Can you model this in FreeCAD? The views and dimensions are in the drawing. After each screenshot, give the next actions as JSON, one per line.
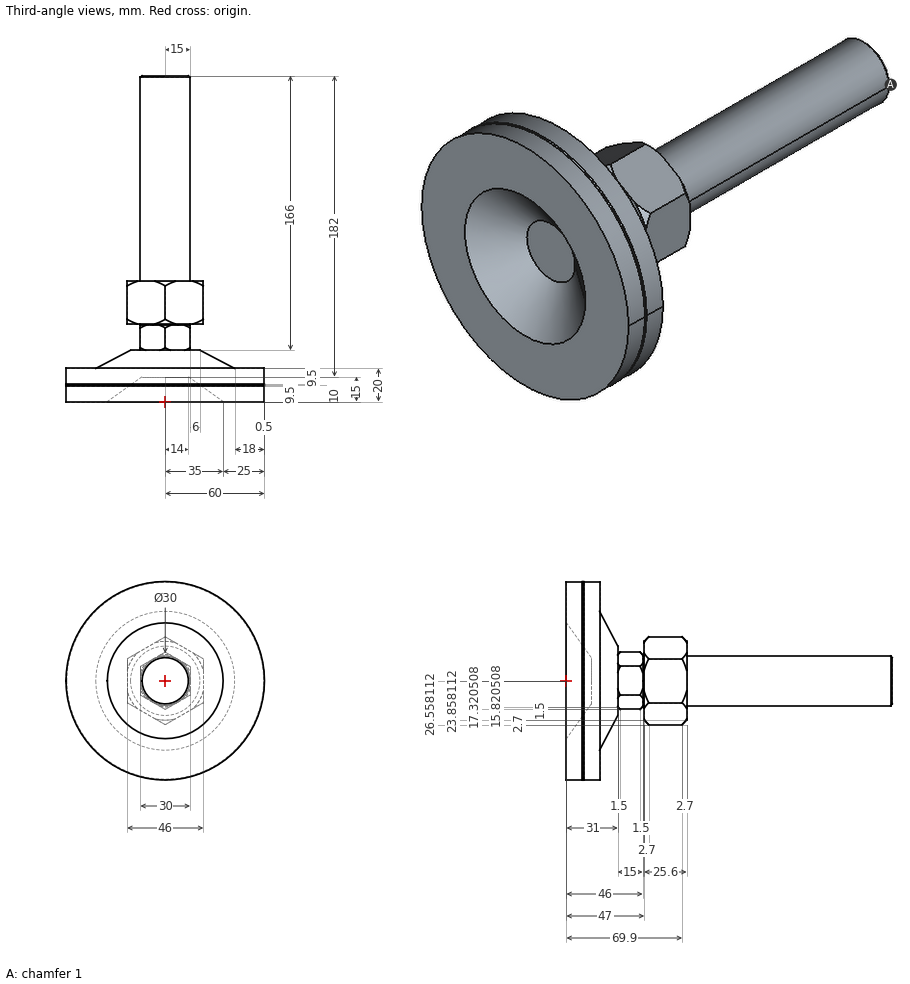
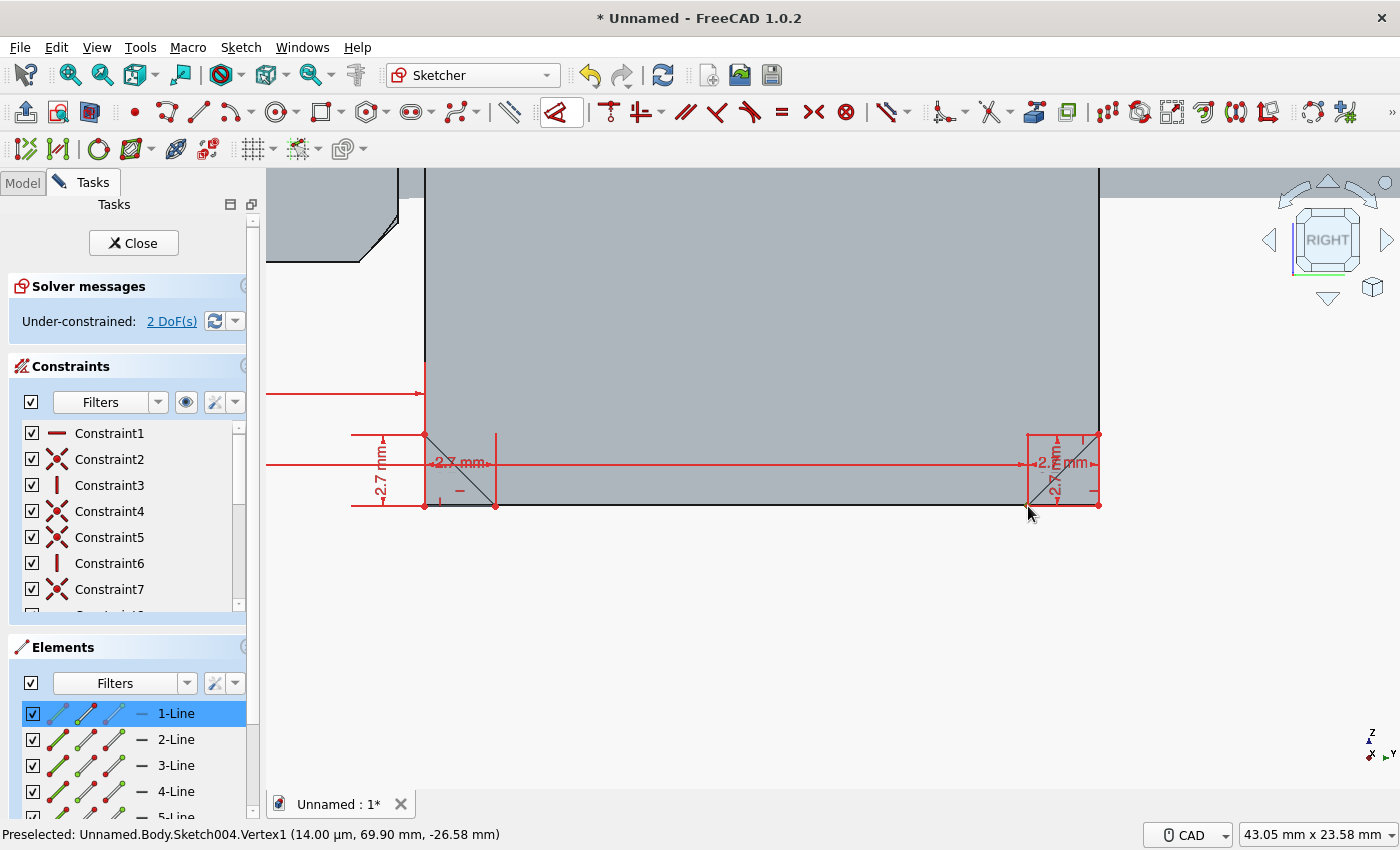
{"action": "key", "text": "i"}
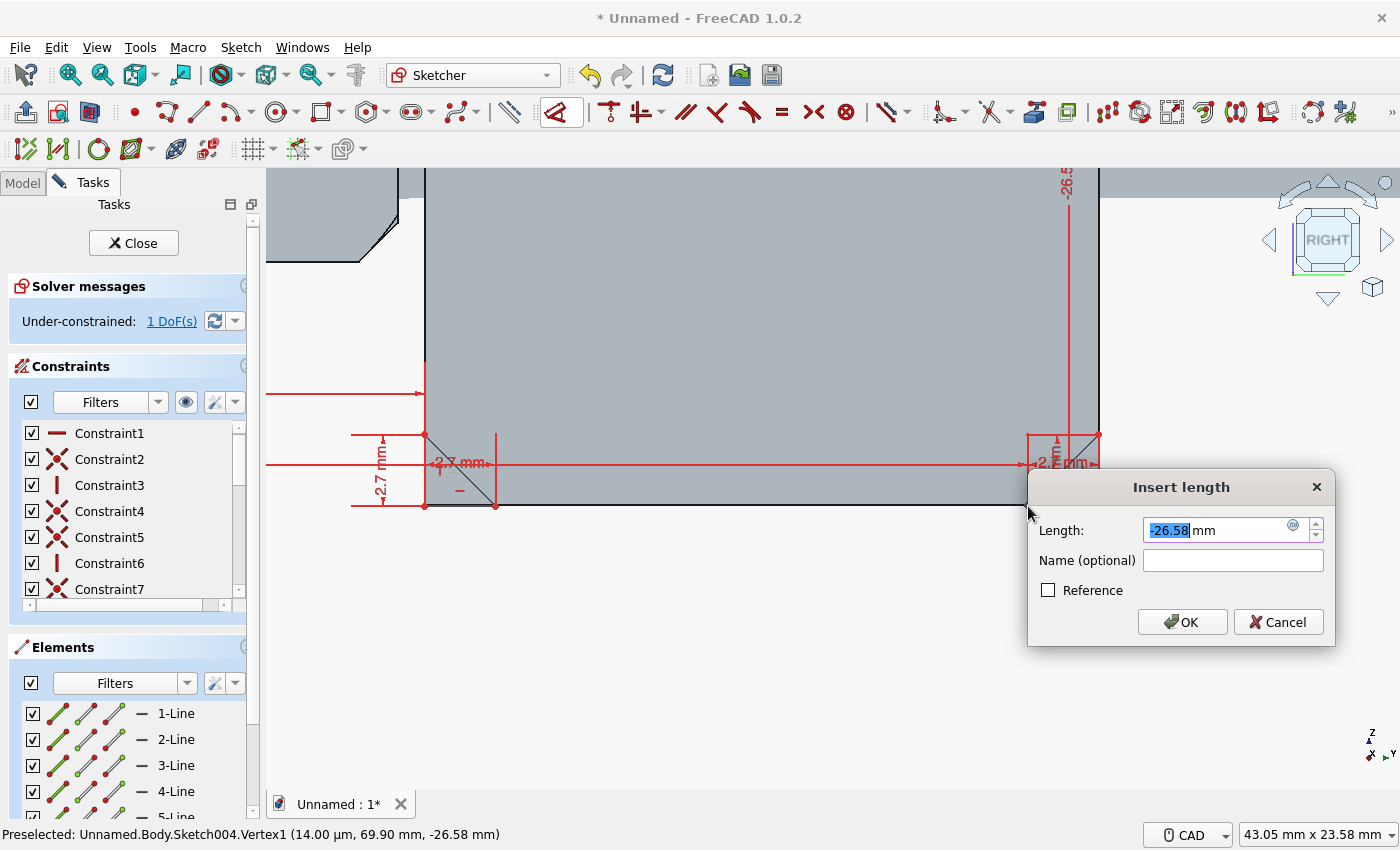
{"action": "type", "text": "-26.558112"}
{"action": "key", "text": "Return"}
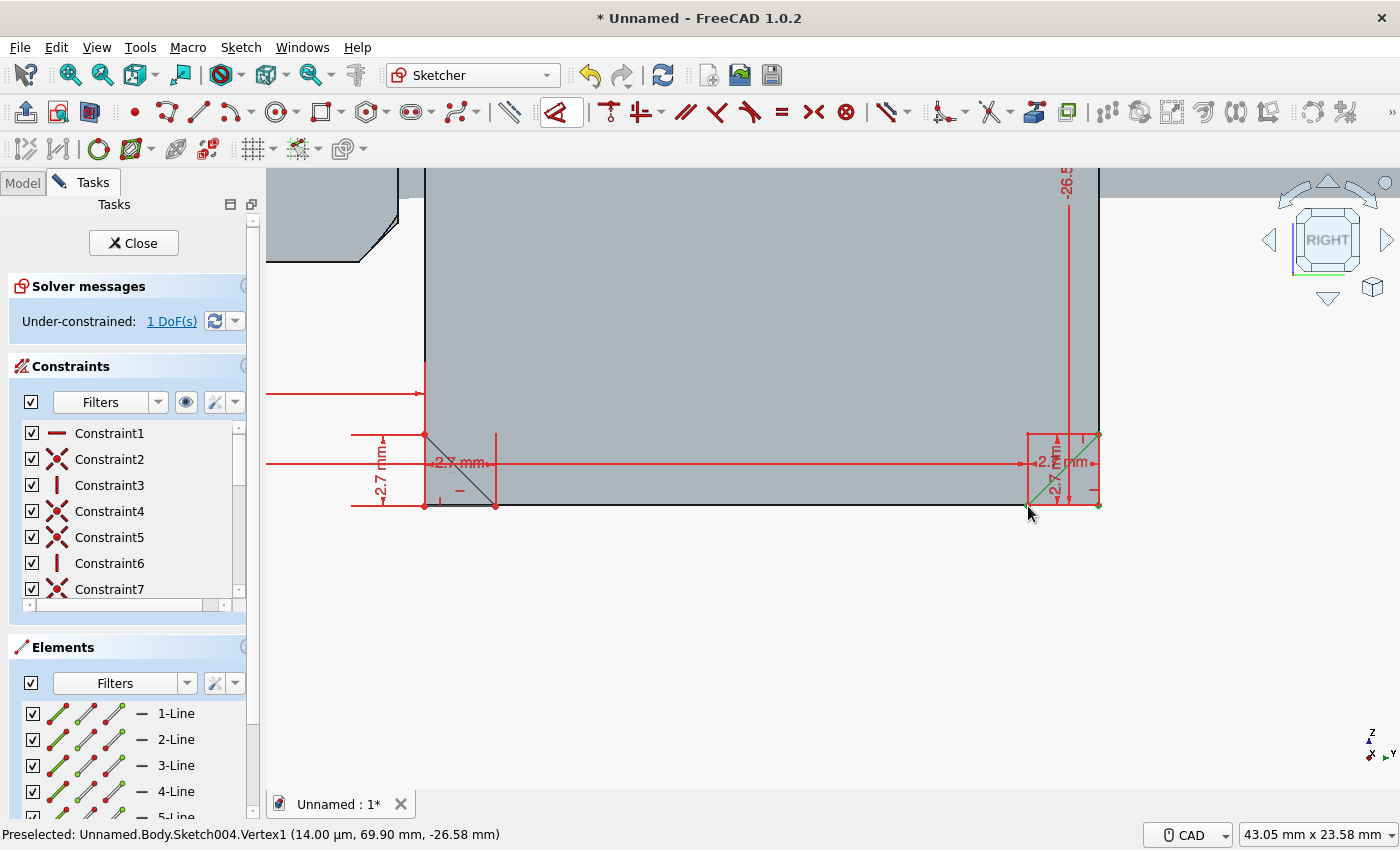
{"action": "left_click", "coordinate": [425, 435]}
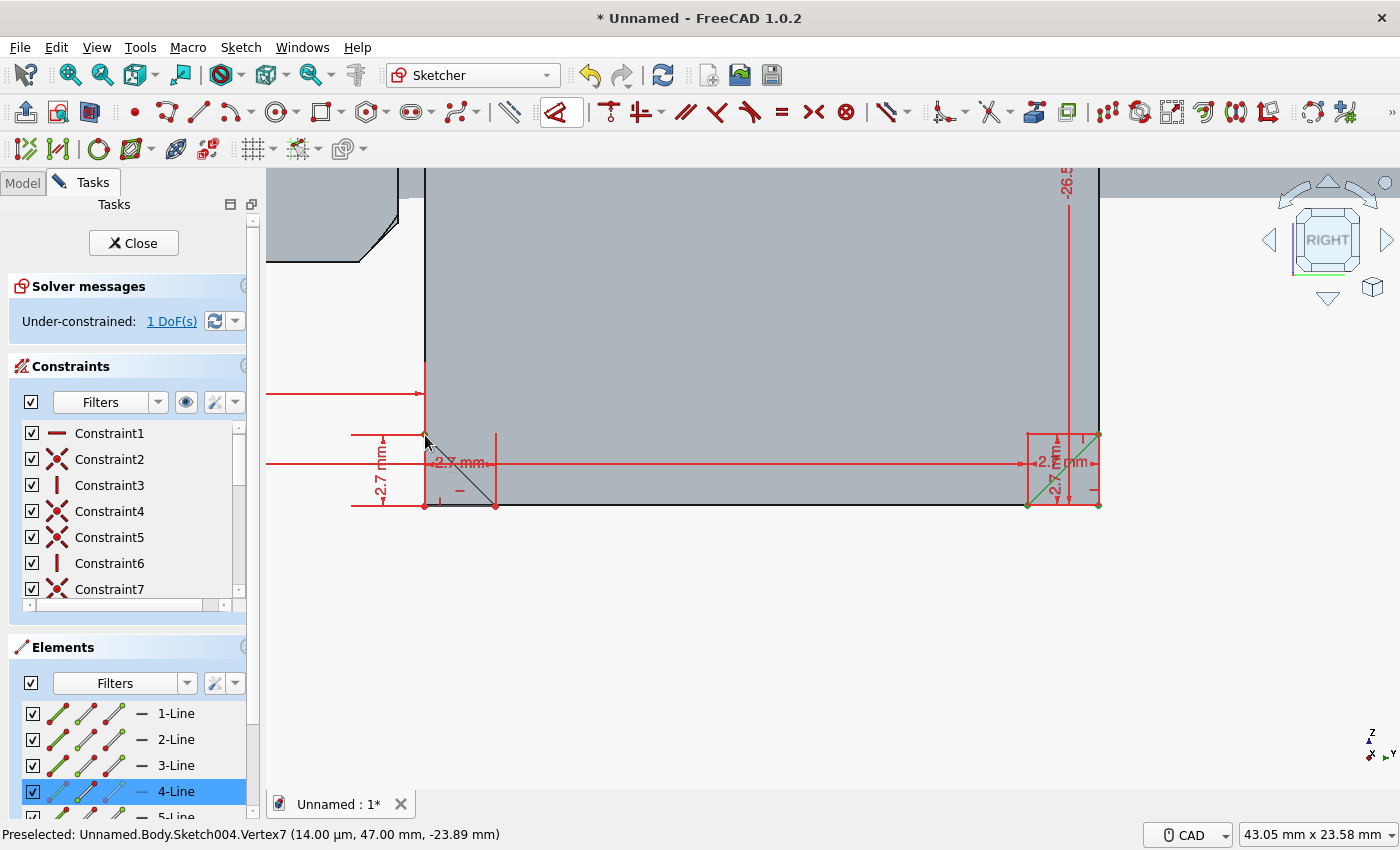
{"action": "key", "text": "i"}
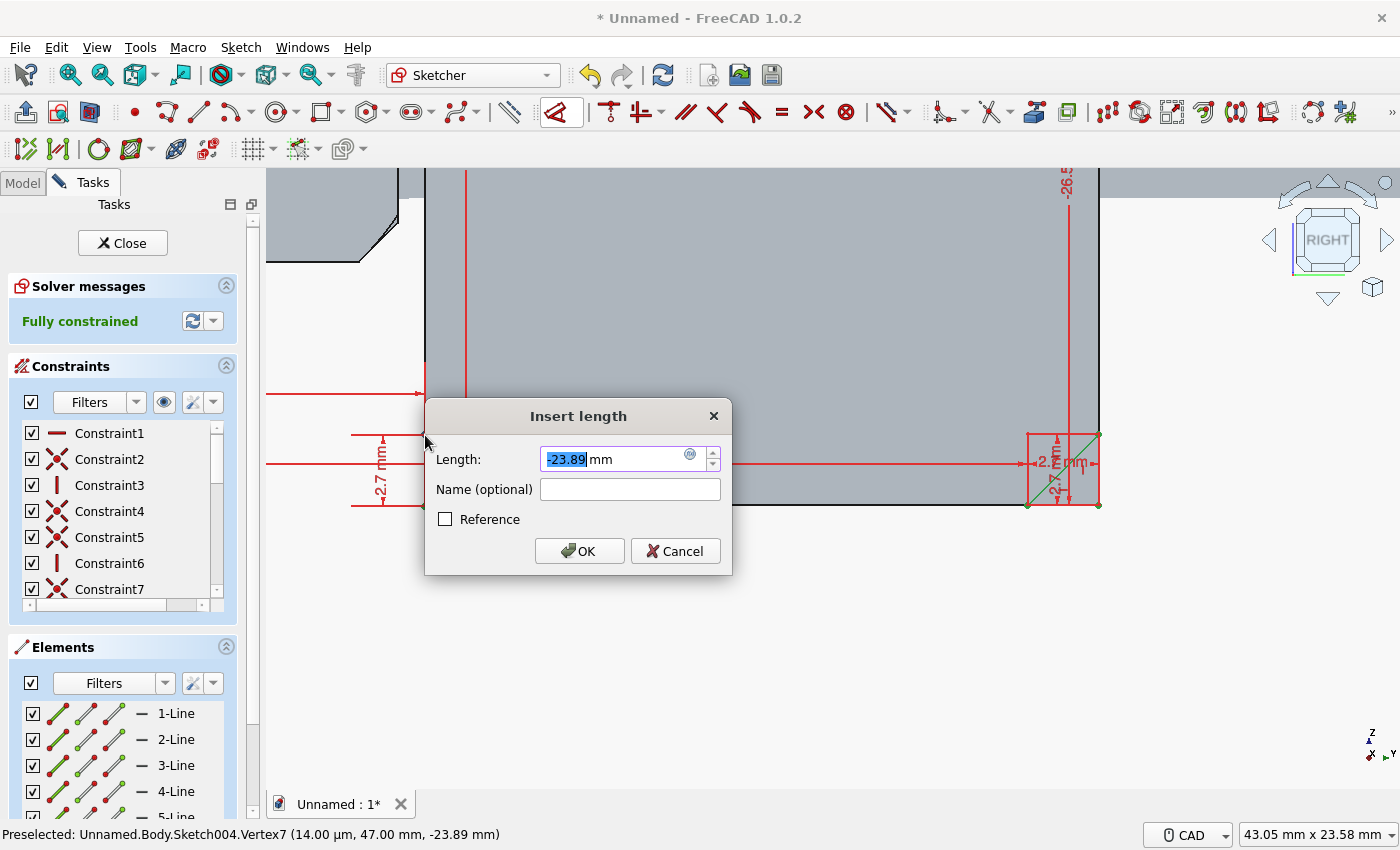
{"action": "type", "text": "-23.858112"}
{"action": "key", "text": "Return"}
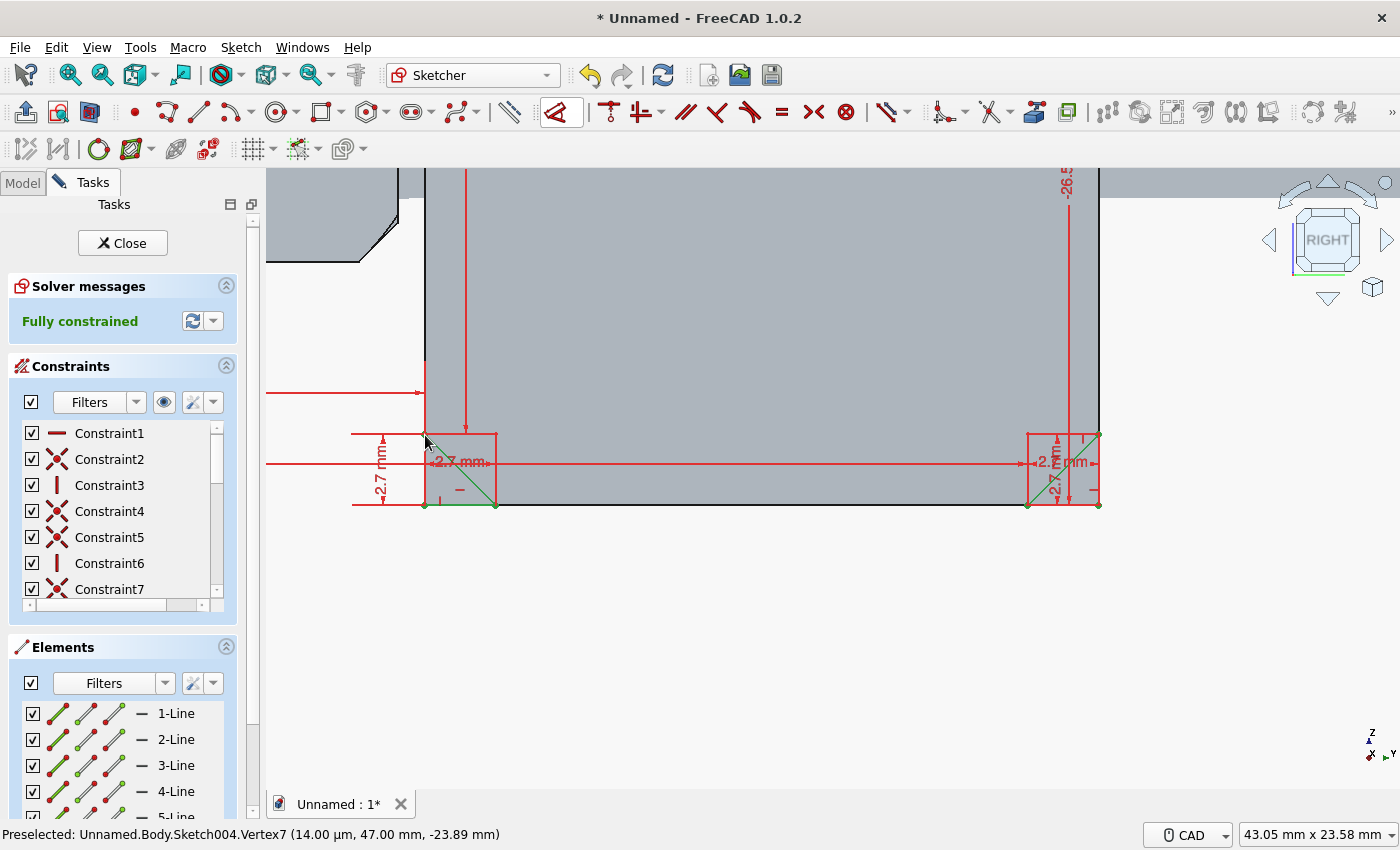
{"action": "left_click", "coordinate": [123, 243]}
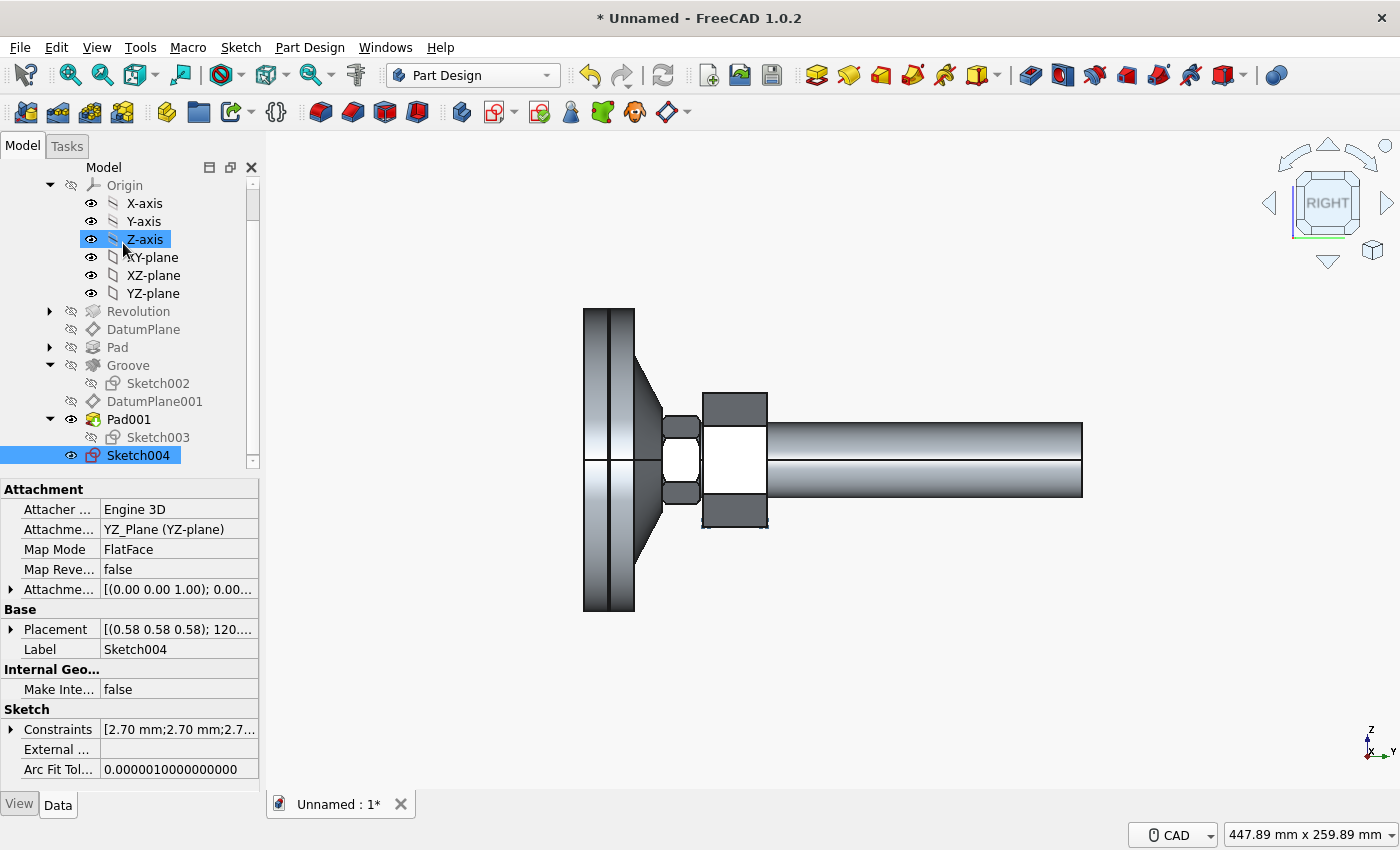
{"action": "left_click", "coordinate": [1096, 76]}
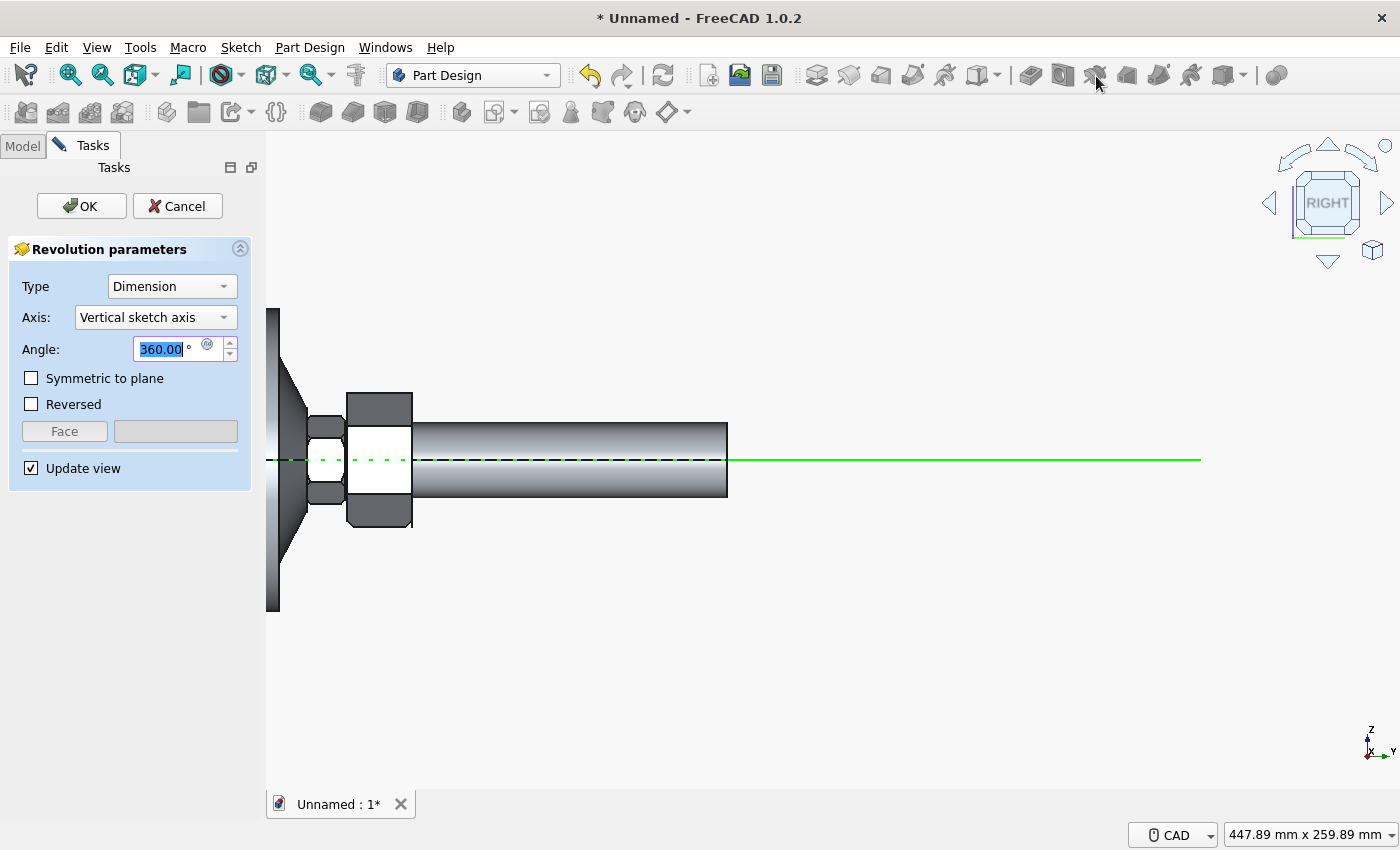
{"action": "left_click", "coordinate": [156, 318]}